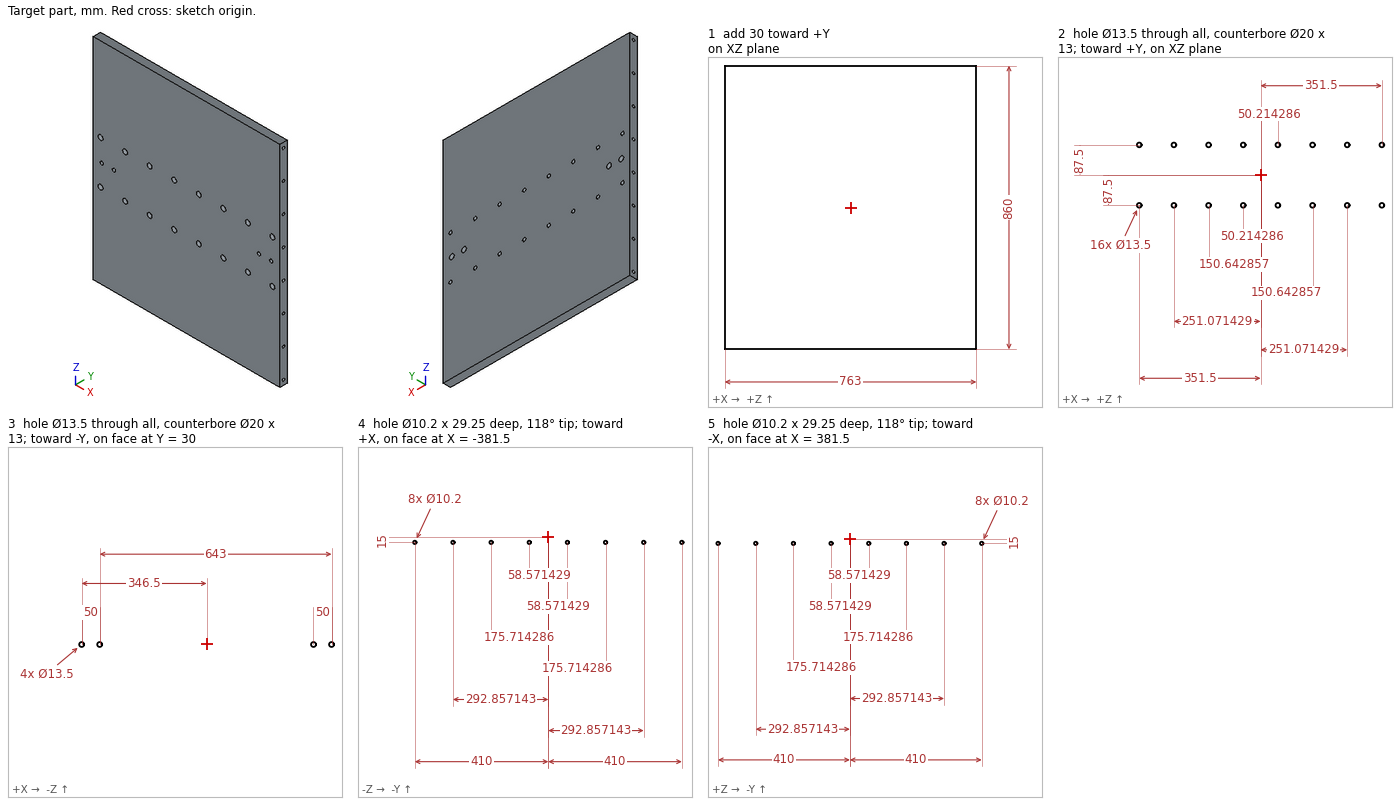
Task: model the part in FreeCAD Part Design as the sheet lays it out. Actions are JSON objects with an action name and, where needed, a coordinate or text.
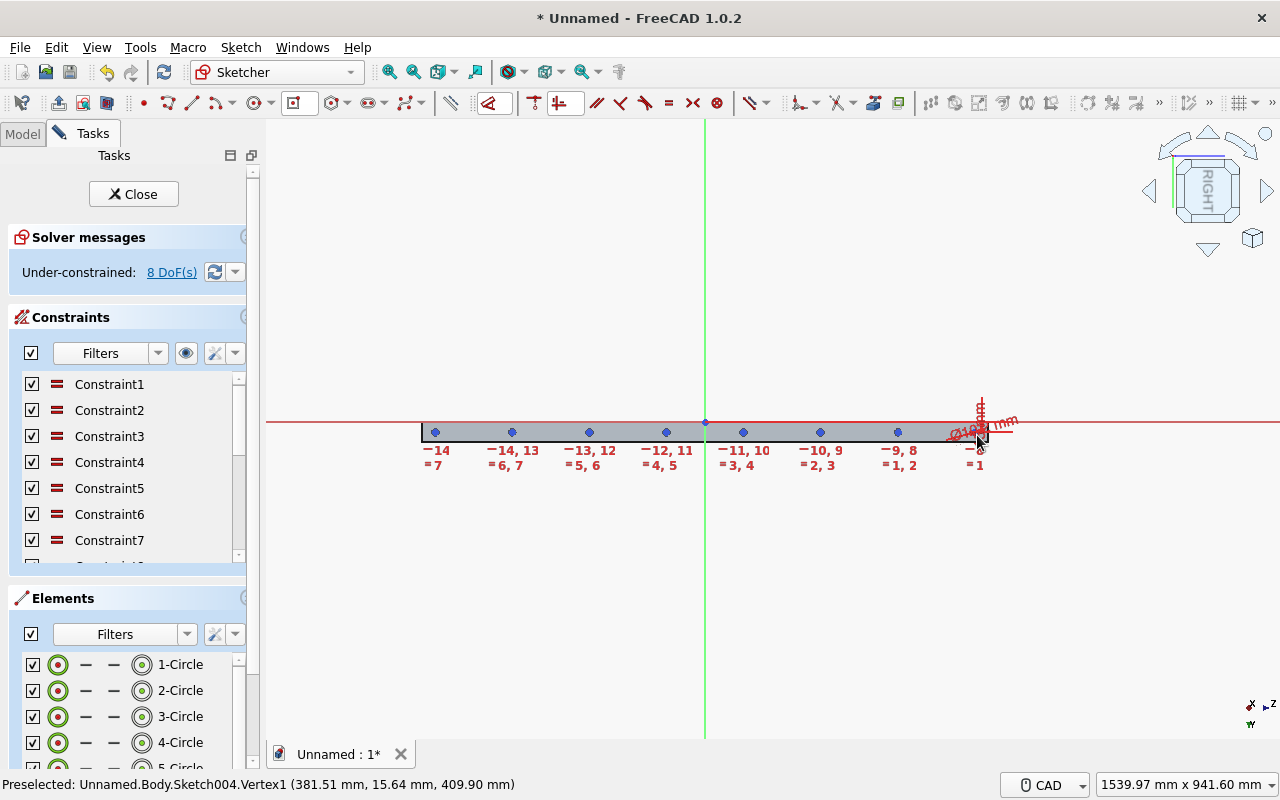
{"action": "left_click", "coordinate": [975, 432]}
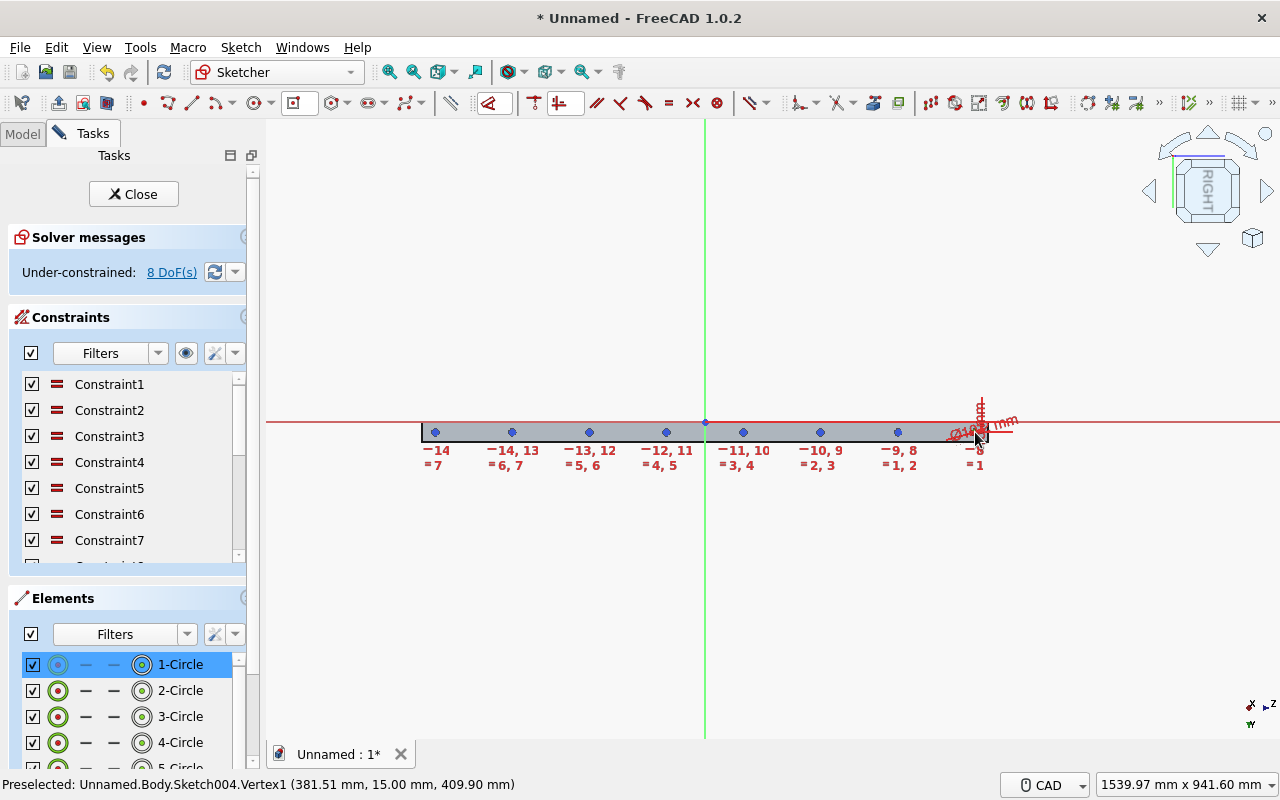
{"action": "left_click", "coordinate": [506, 104]}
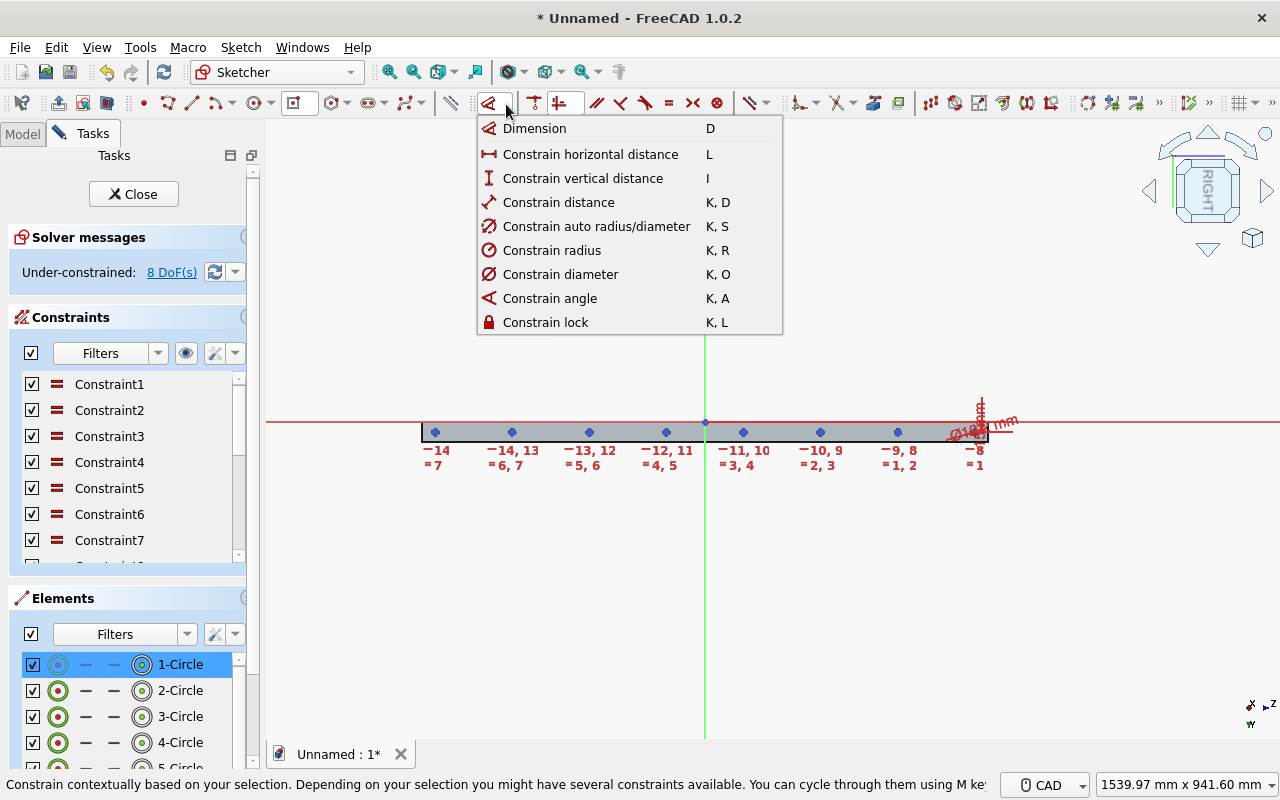
{"action": "left_click", "coordinate": [630, 154]}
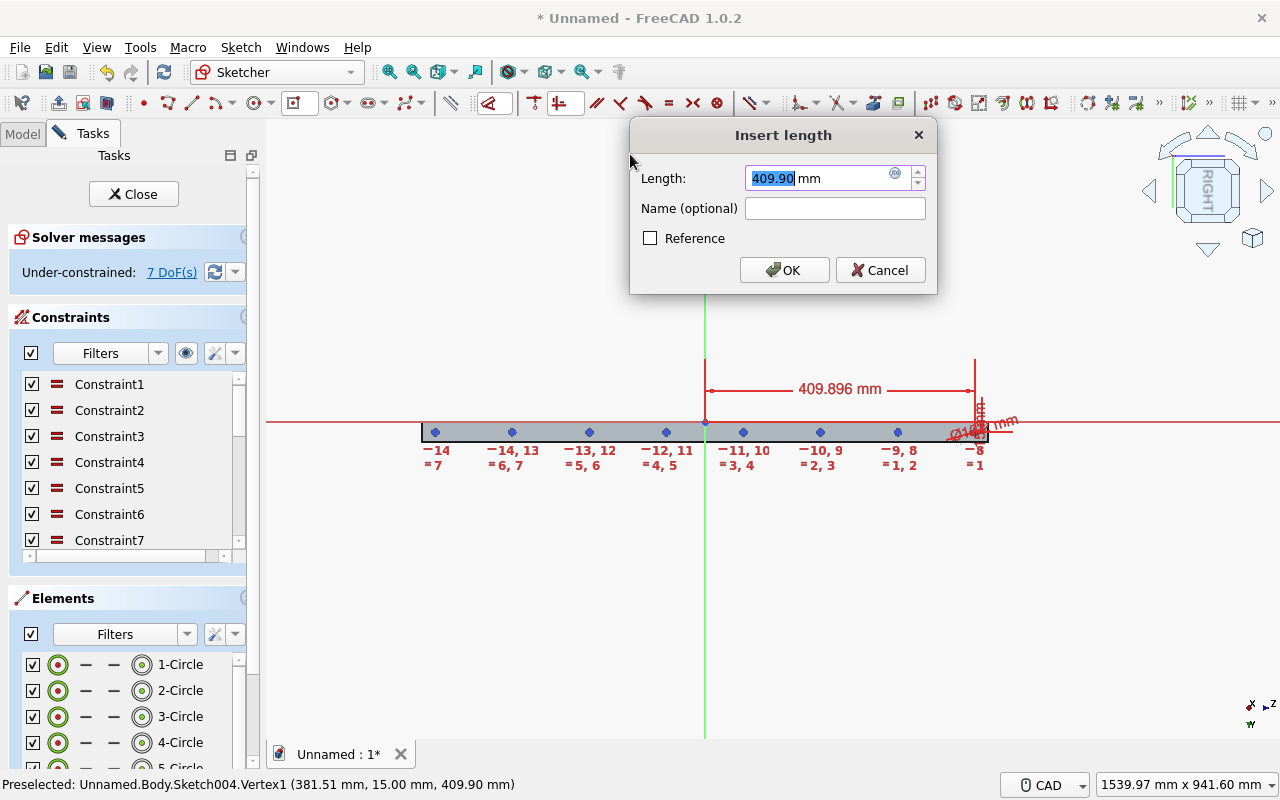
{"action": "type", "text": "410"}
{"action": "key", "text": "Return"}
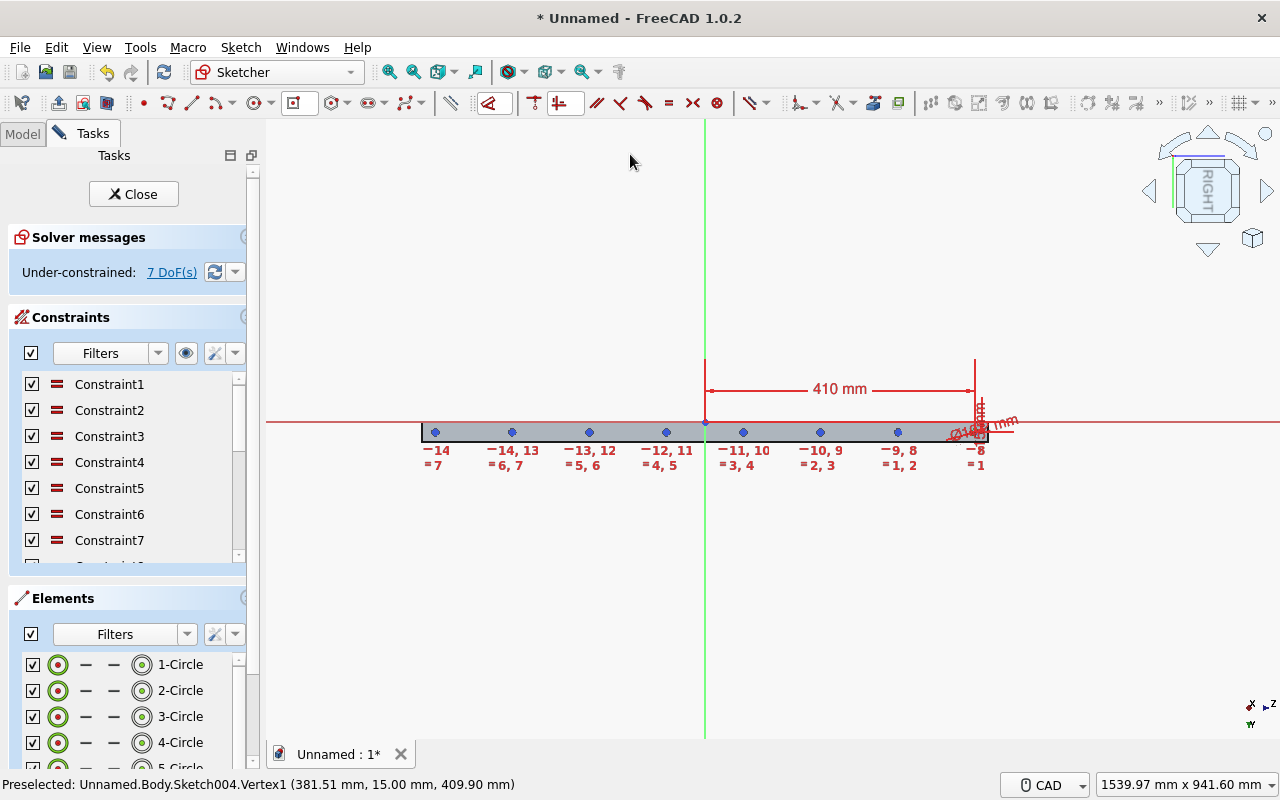
{"action": "left_click", "coordinate": [435, 432]}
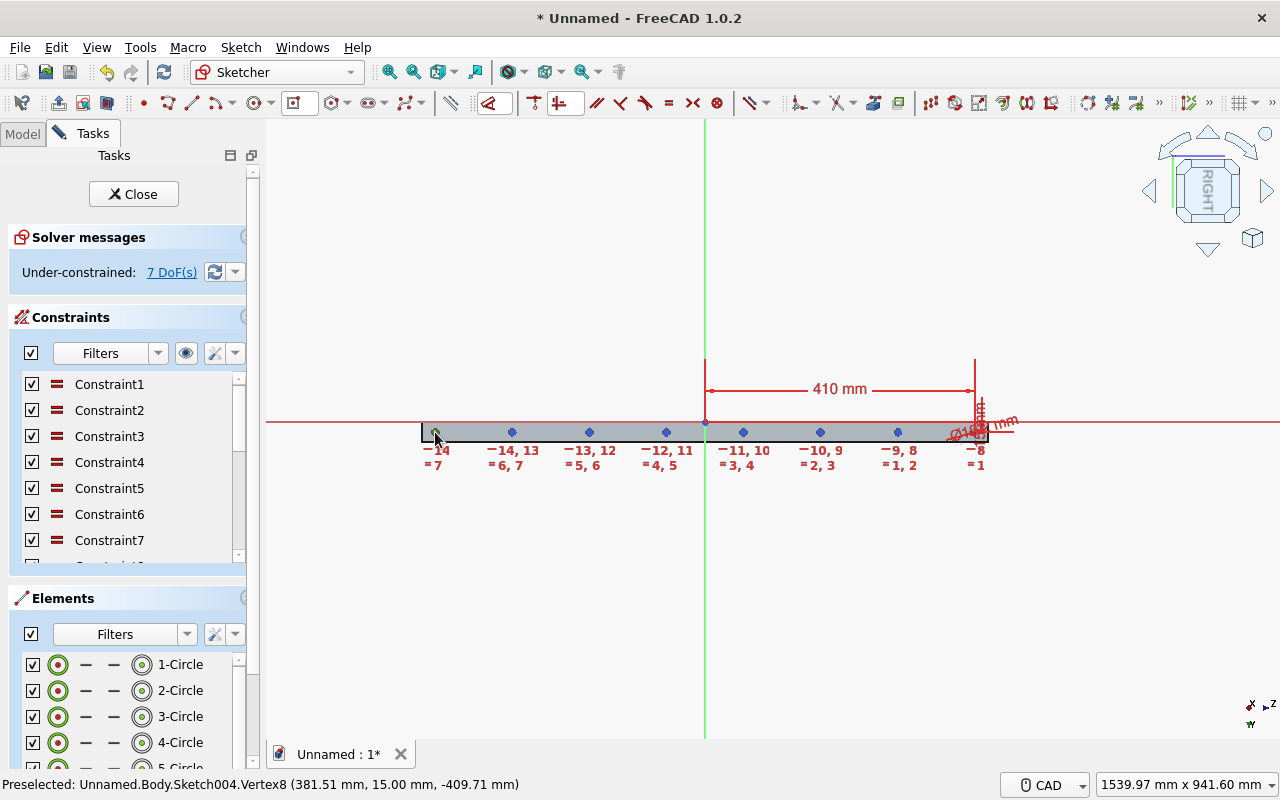
{"action": "key", "text": "l"}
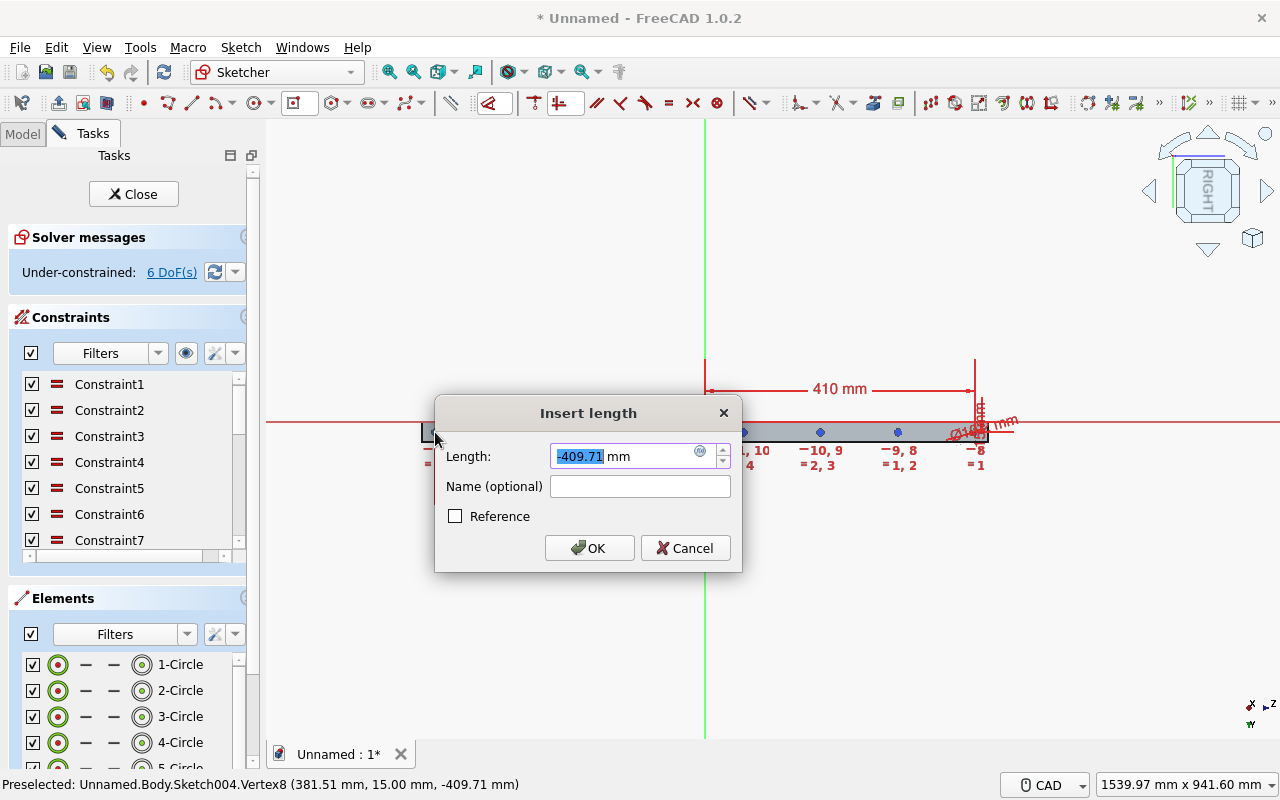
{"action": "type", "text": "-410"}
{"action": "key", "text": "Return"}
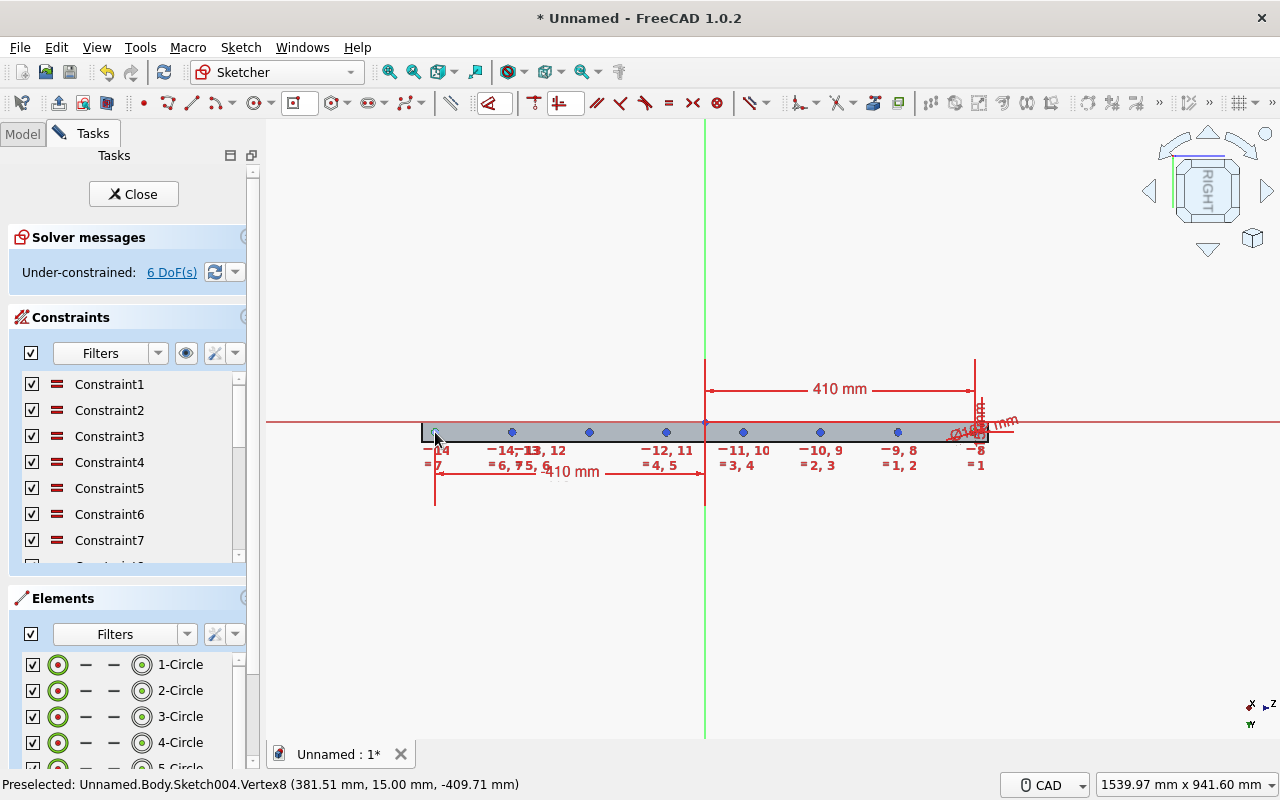
{"action": "left_click", "coordinate": [743, 432]}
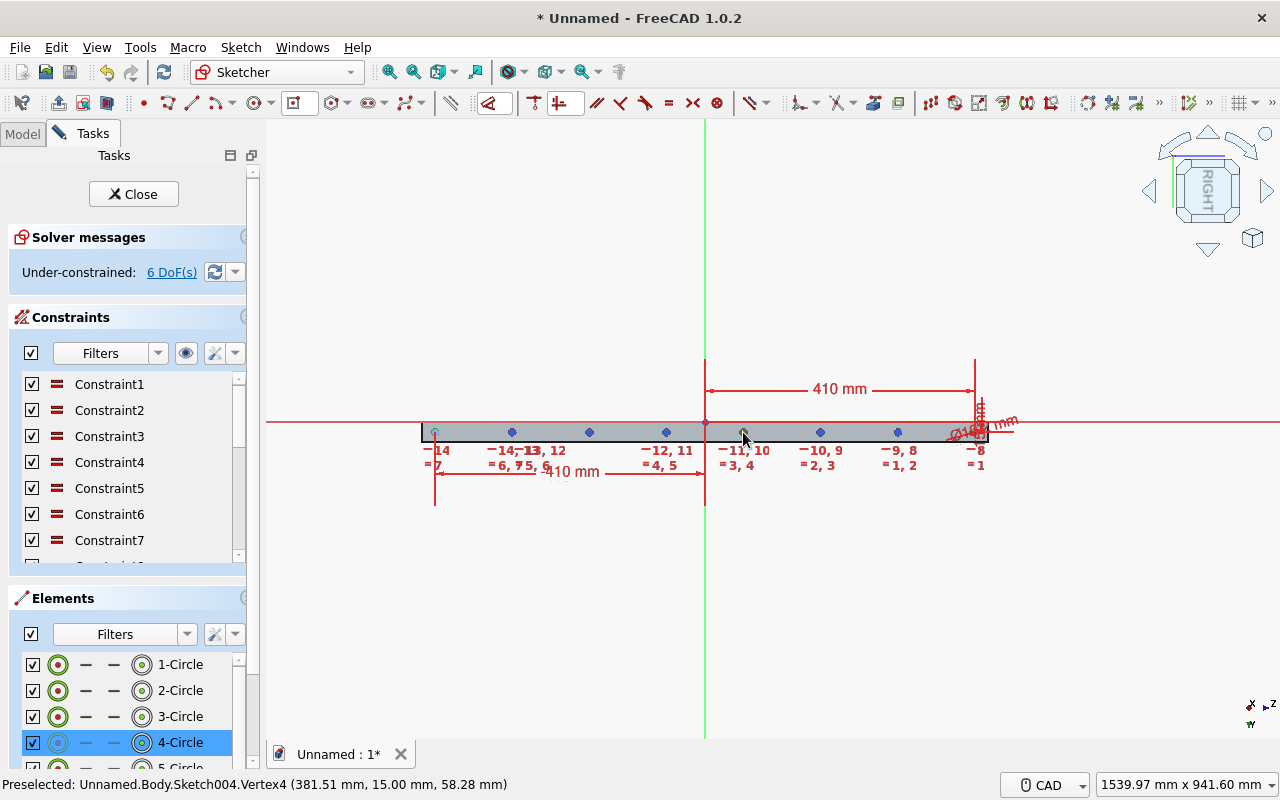
{"action": "key", "text": "l"}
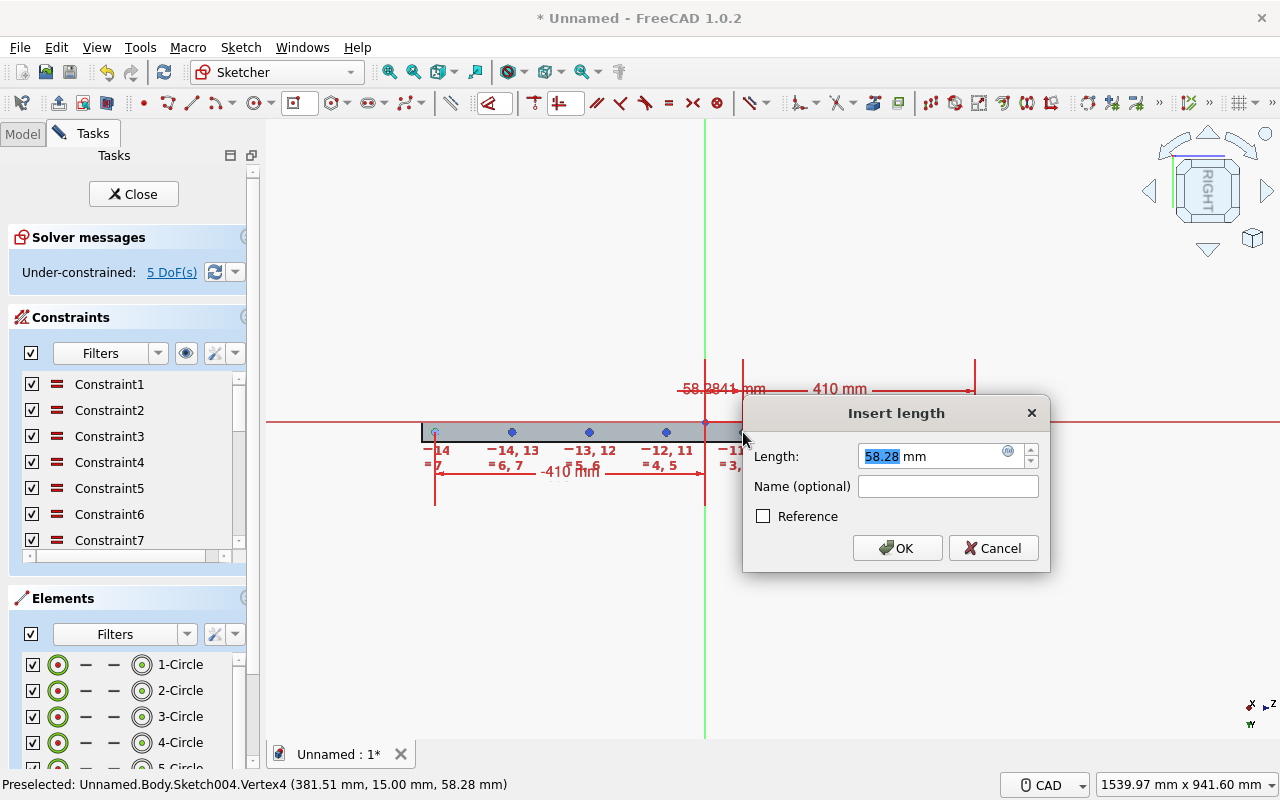
{"action": "type", "text": "58.571429"}
{"action": "key", "text": "Return"}